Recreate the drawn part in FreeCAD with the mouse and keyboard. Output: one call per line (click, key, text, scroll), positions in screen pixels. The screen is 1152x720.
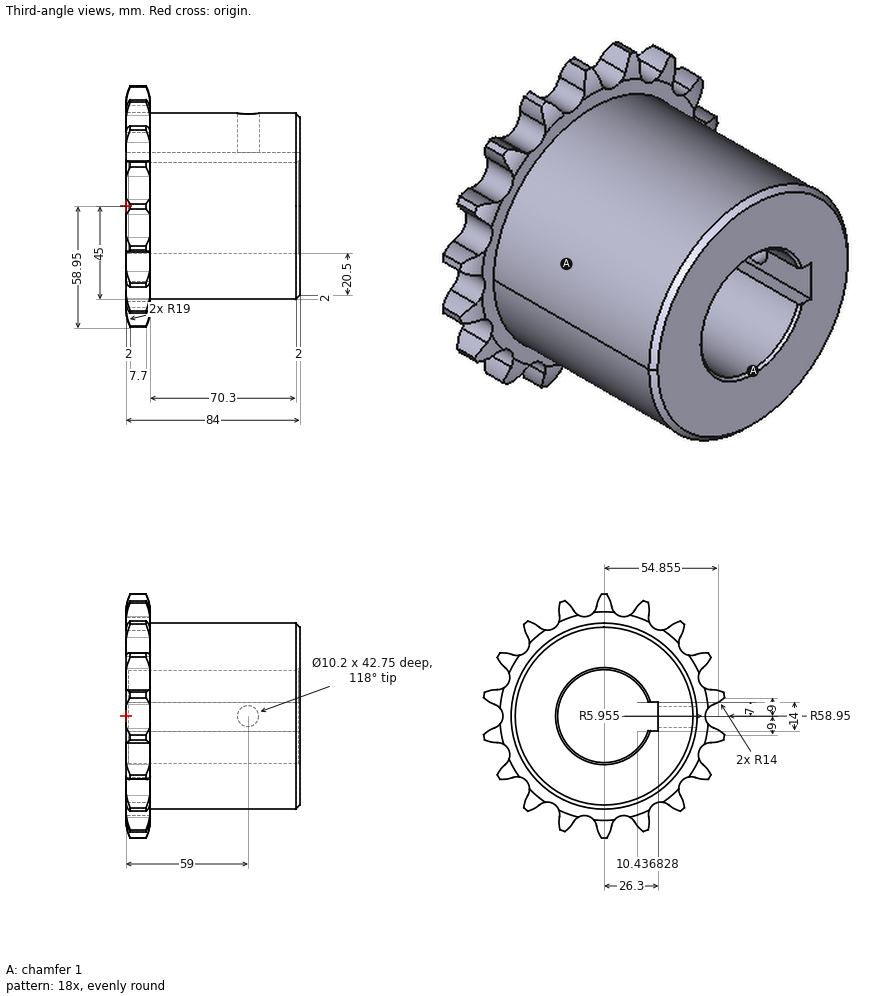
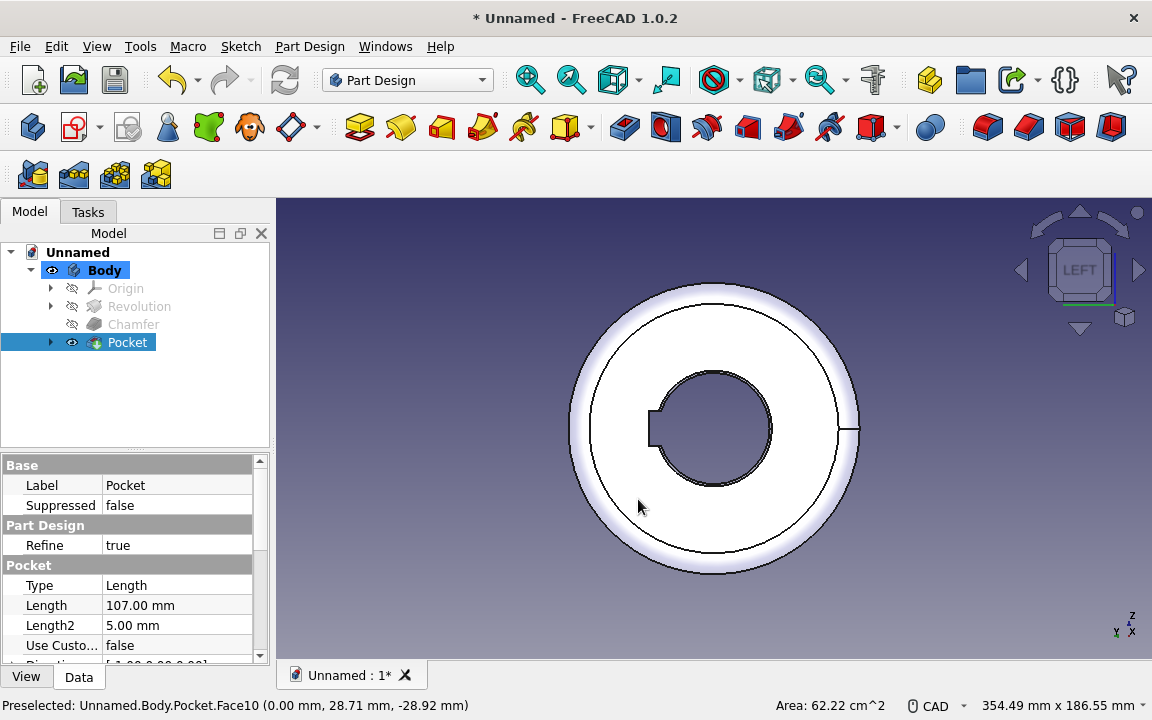
click(74, 128)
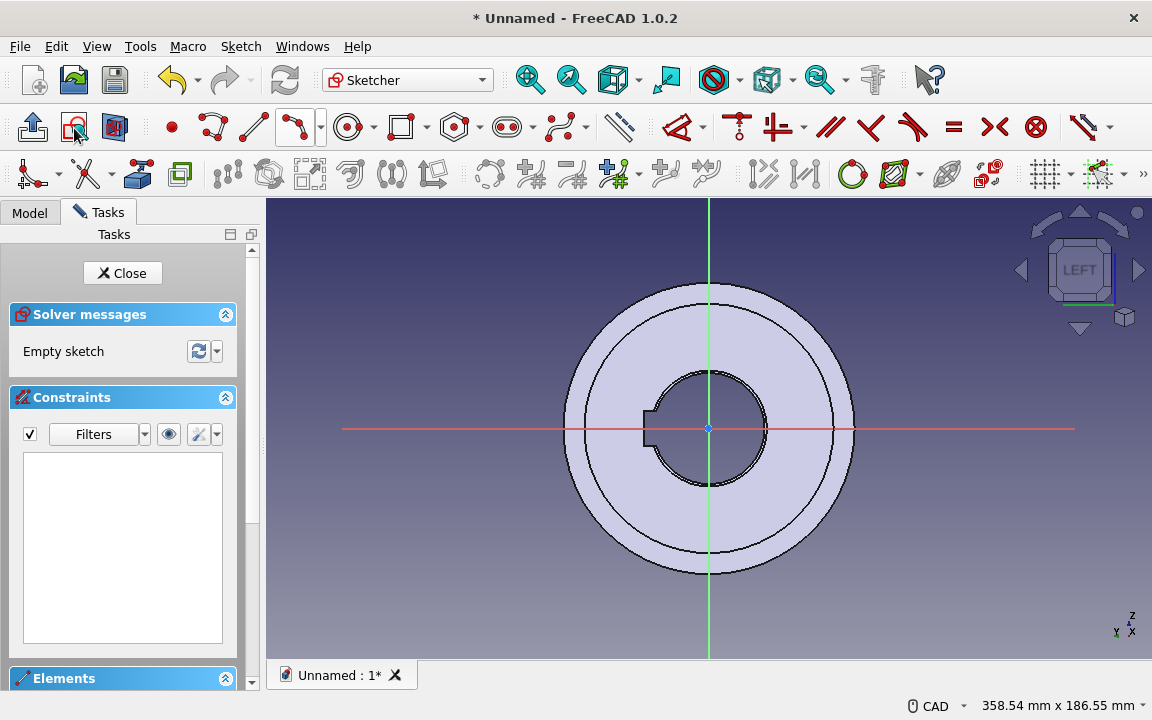
scroll(563, 429, up, 9)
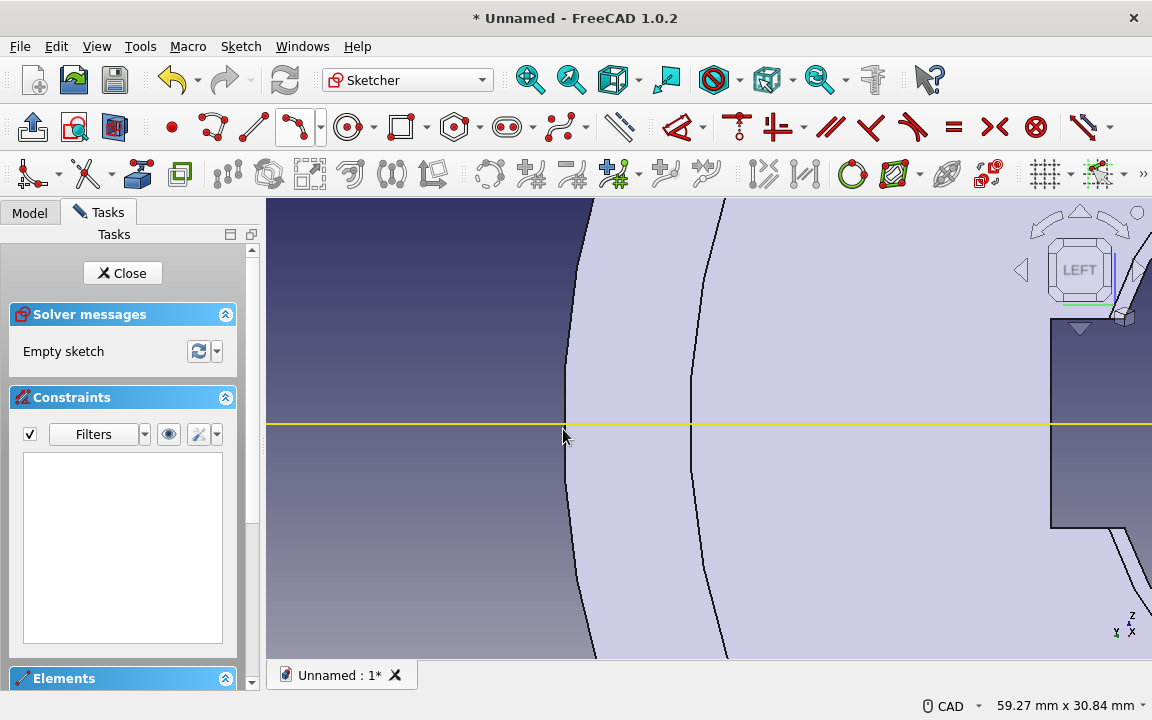
click(294, 128)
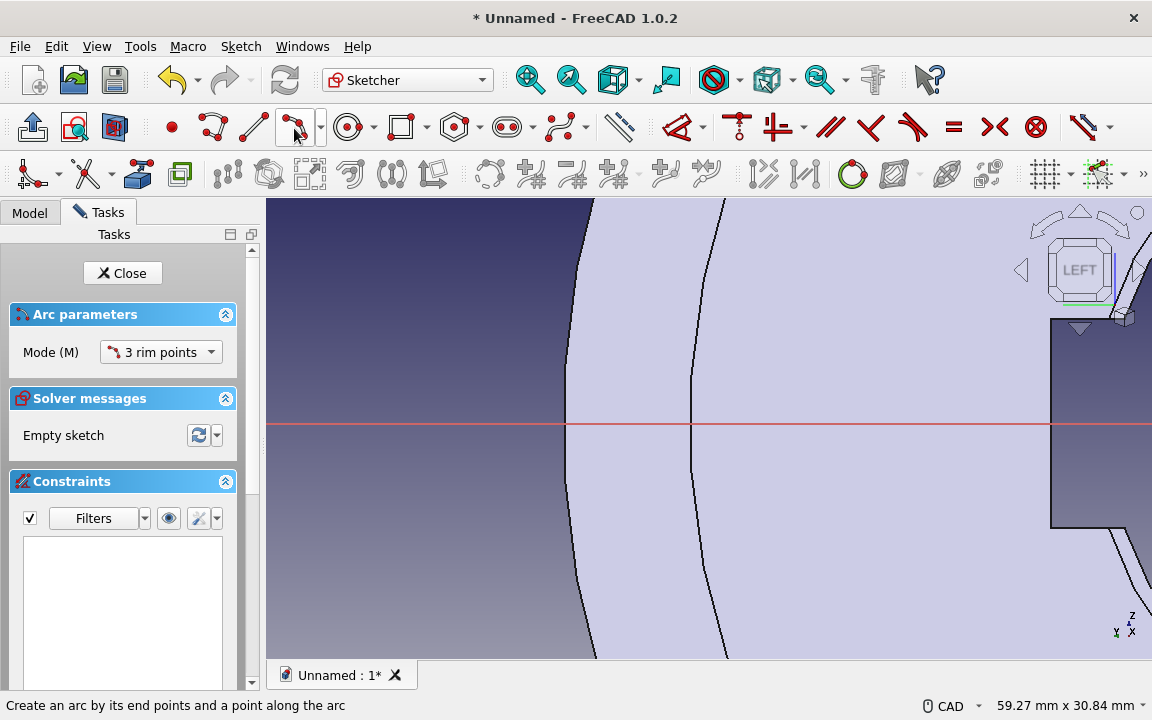
click(653, 508)
click(653, 340)
click(711, 445)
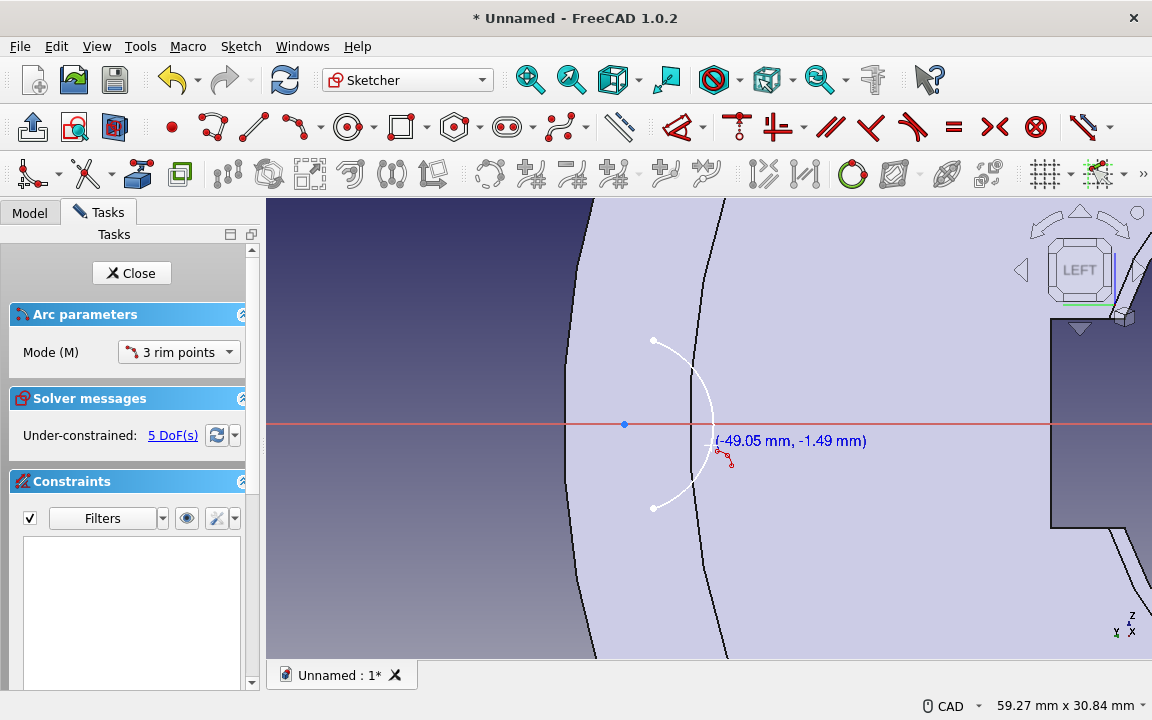
click(653, 341)
click(573, 289)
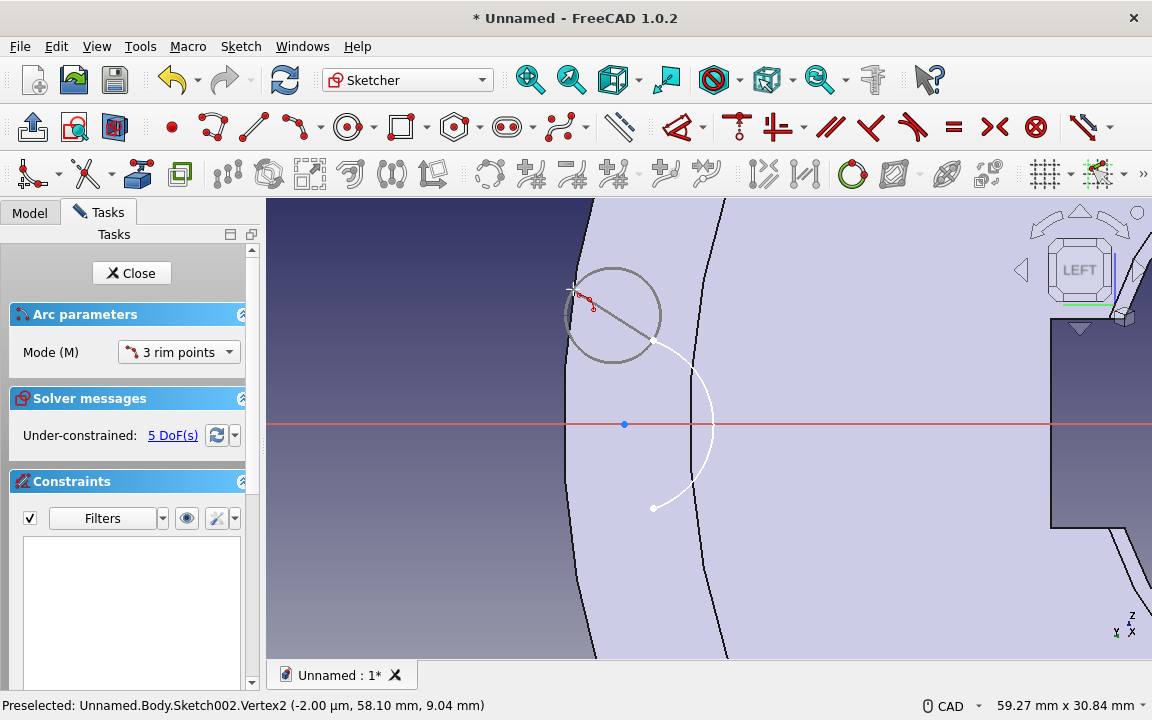
scroll(610, 319, up, 6)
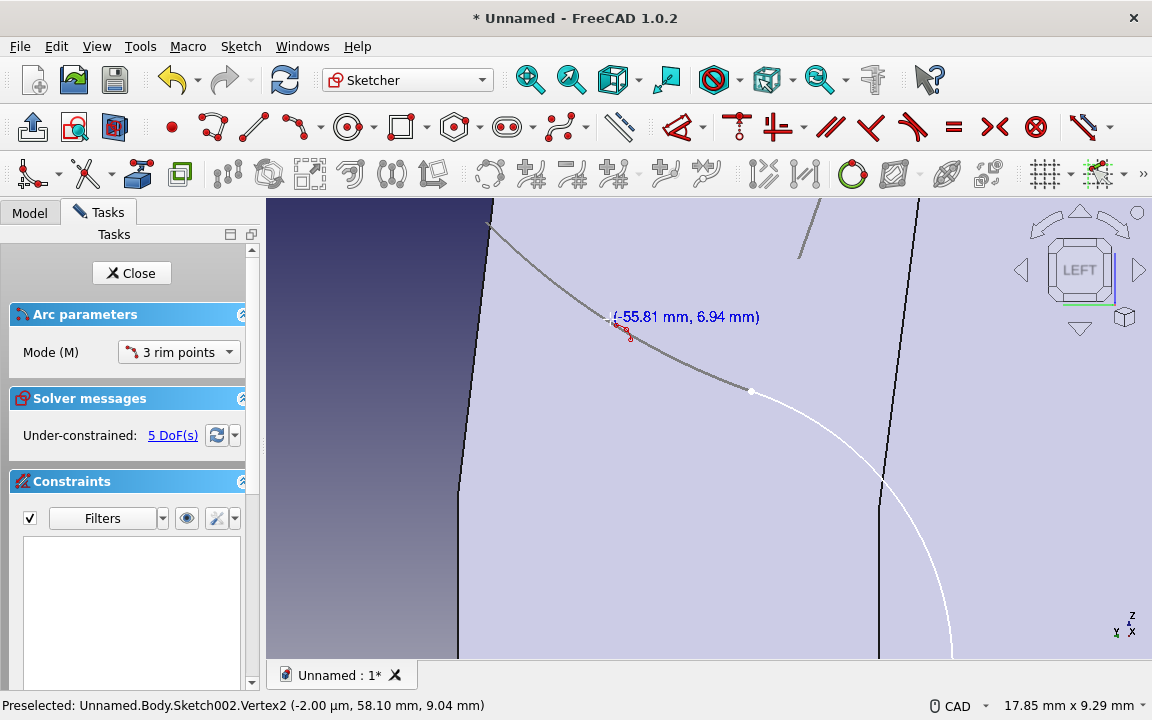
click(611, 318)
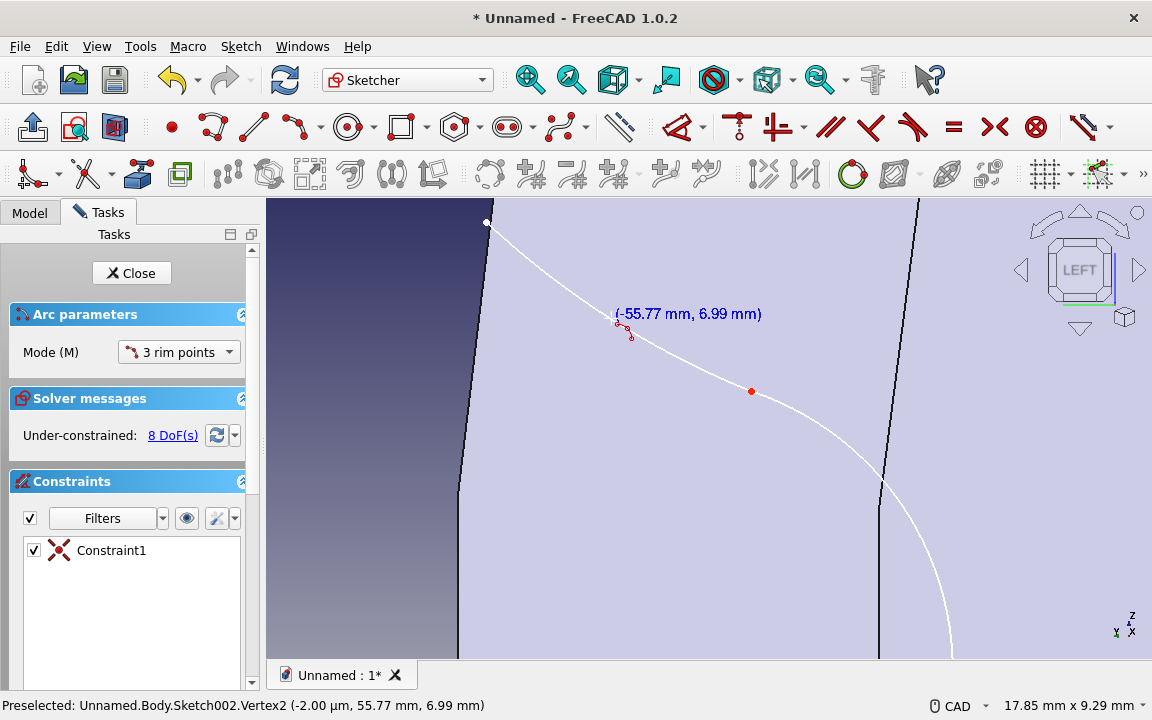
scroll(614, 326, down, 6)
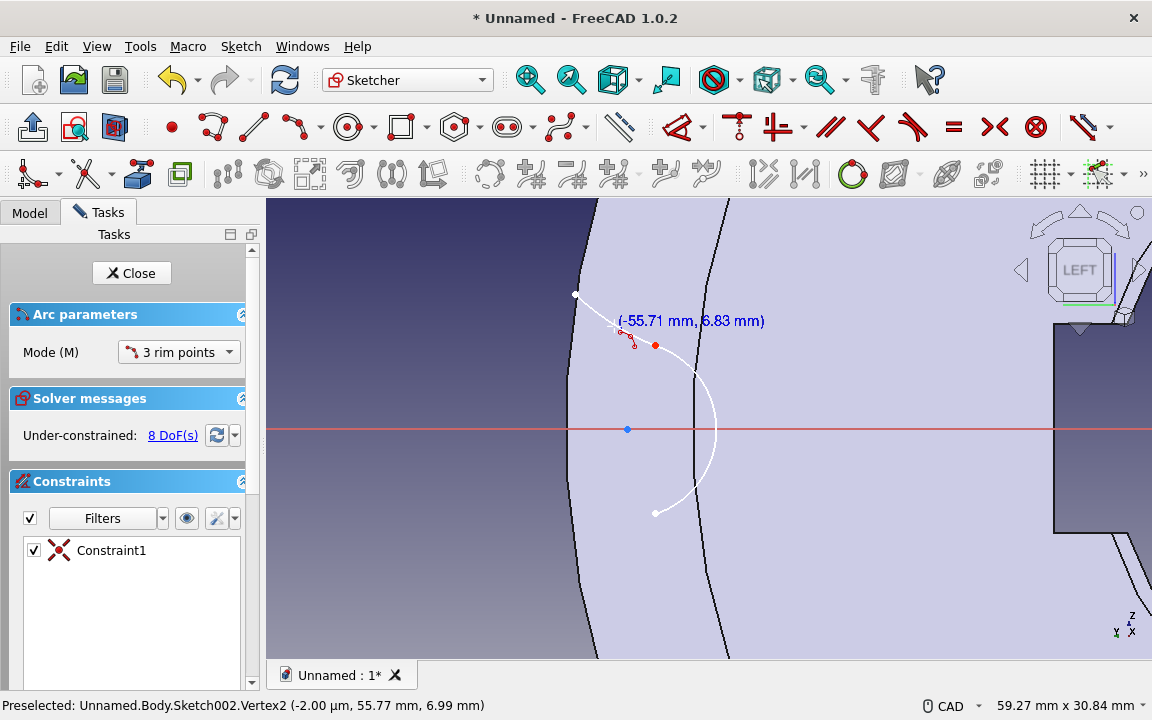
click(576, 295)
click(576, 563)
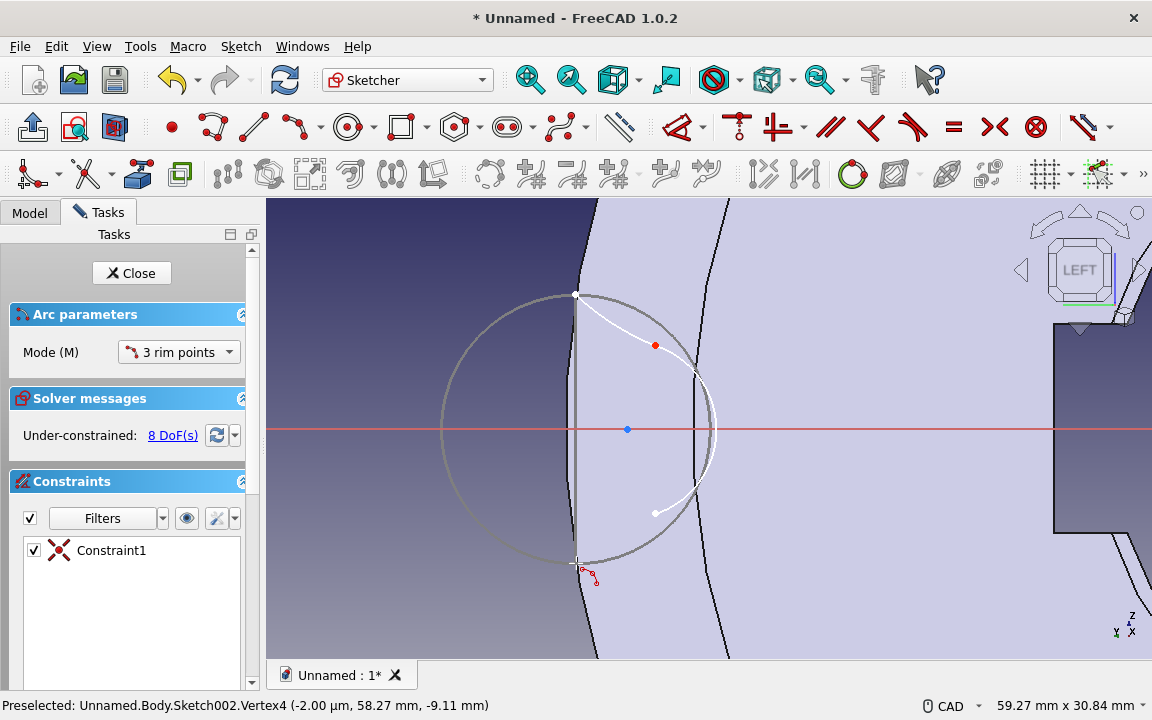
scroll(566, 402, up, 3)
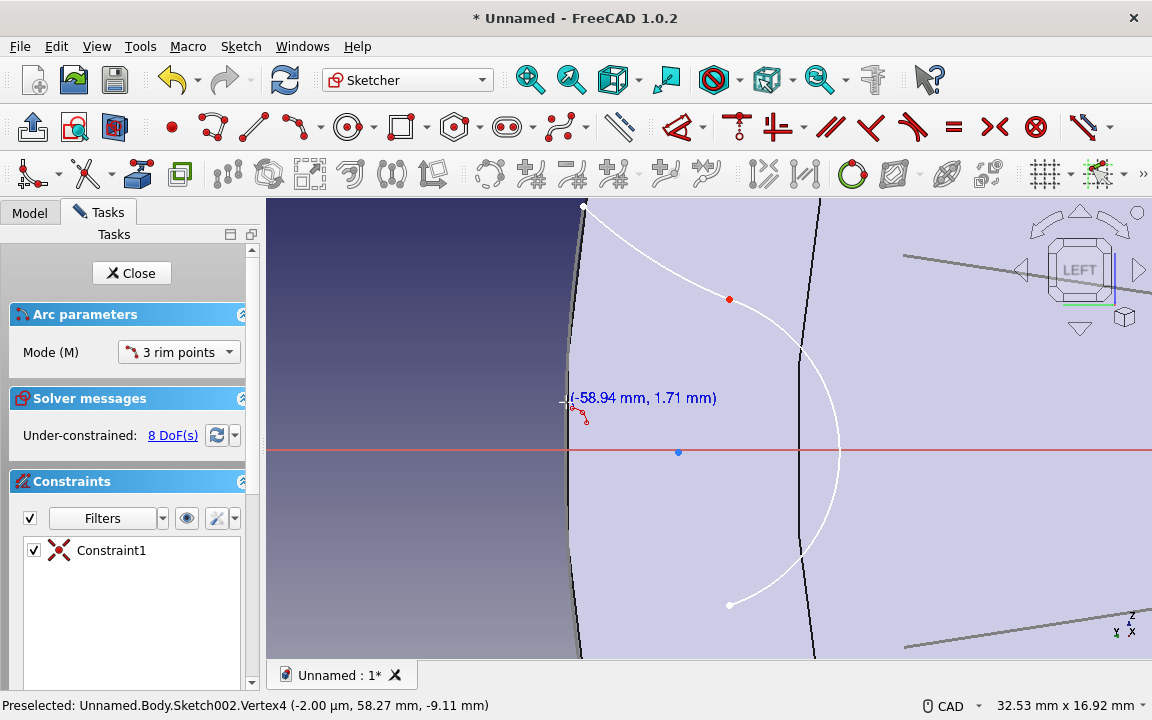
click(566, 401)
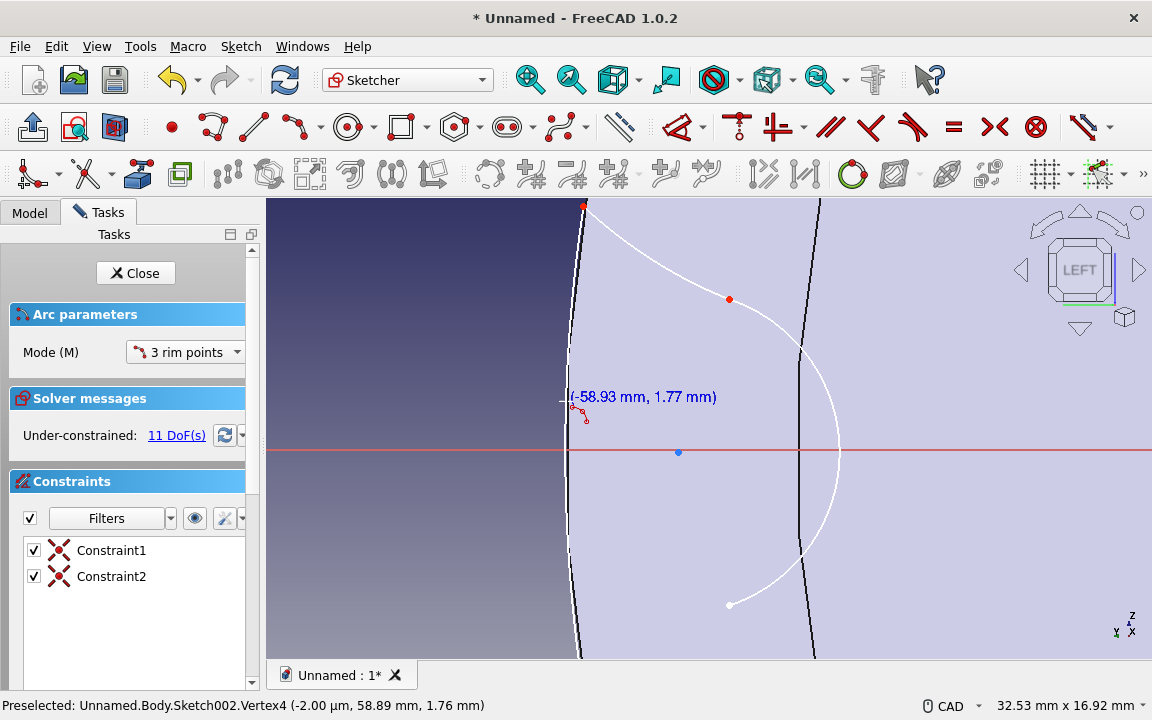
scroll(565, 402, down, 3)